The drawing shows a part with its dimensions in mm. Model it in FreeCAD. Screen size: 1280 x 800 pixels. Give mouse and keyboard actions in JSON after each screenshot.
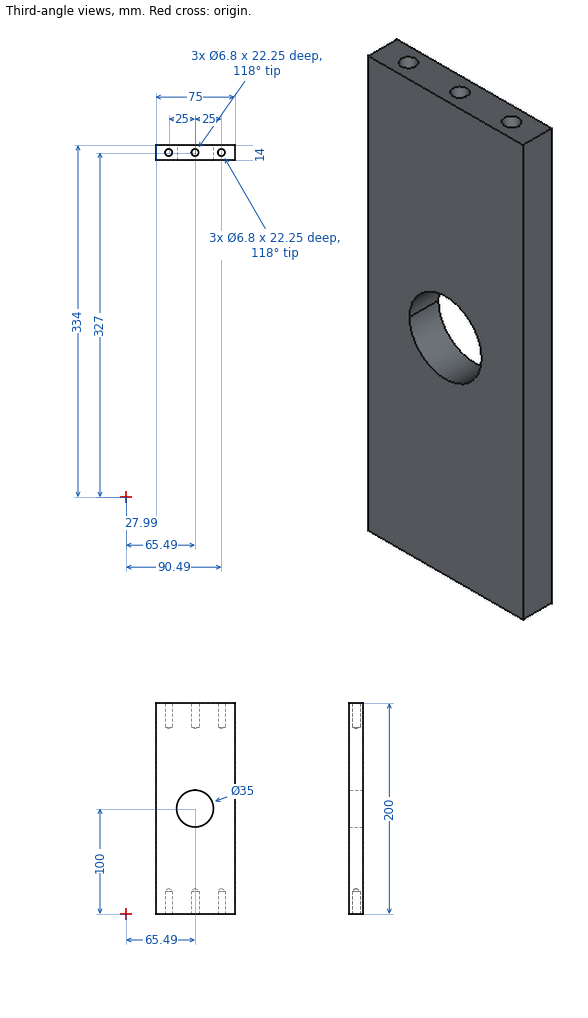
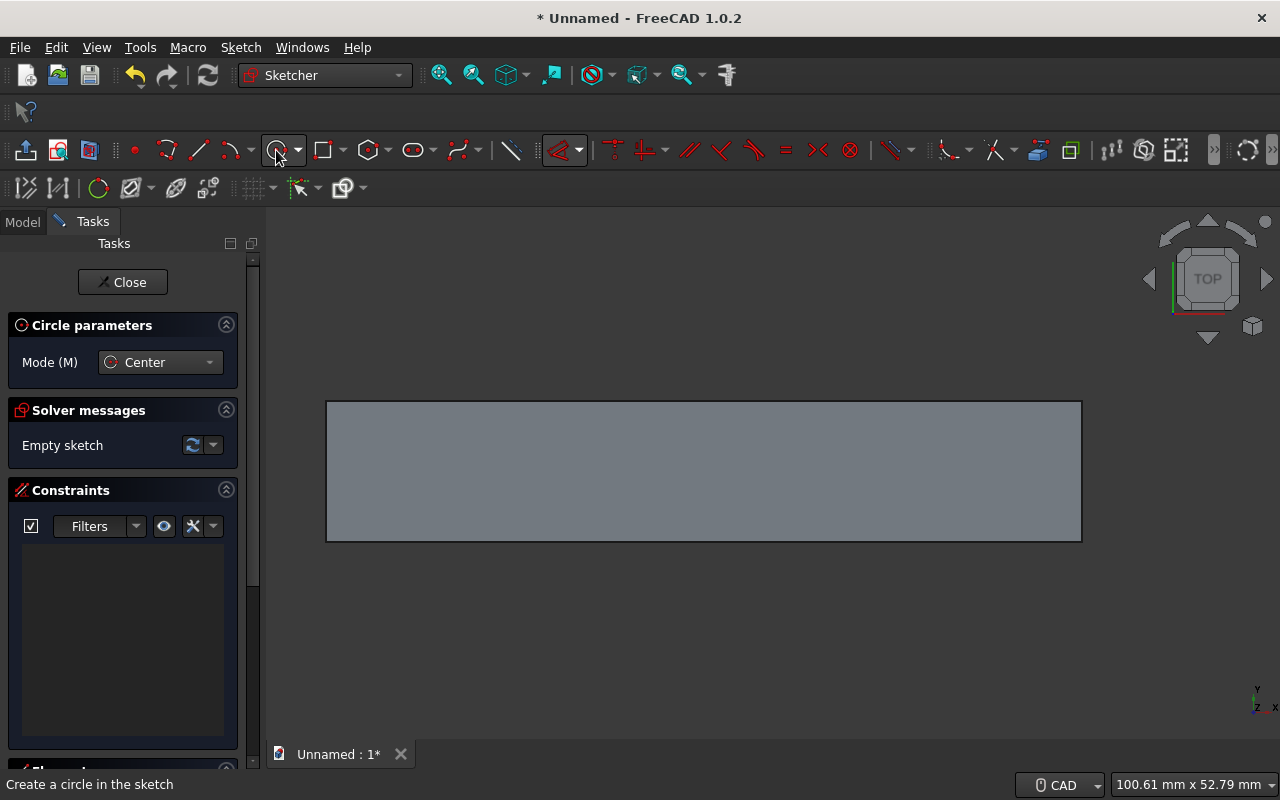
{"action": "left_click", "coordinate": [704, 471]}
{"action": "mouse_move", "coordinate": [728, 447]}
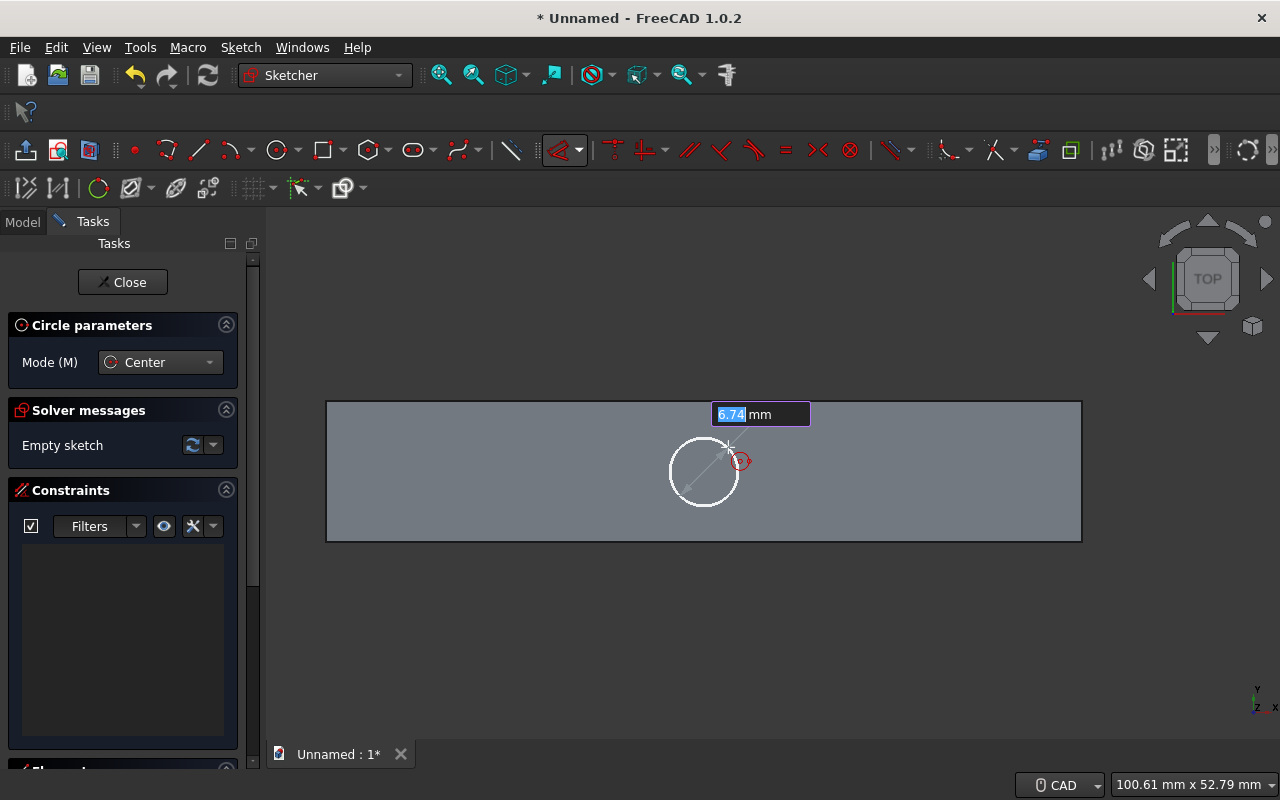
{"action": "type", "text": "6.8"}
{"action": "key", "text": "Return"}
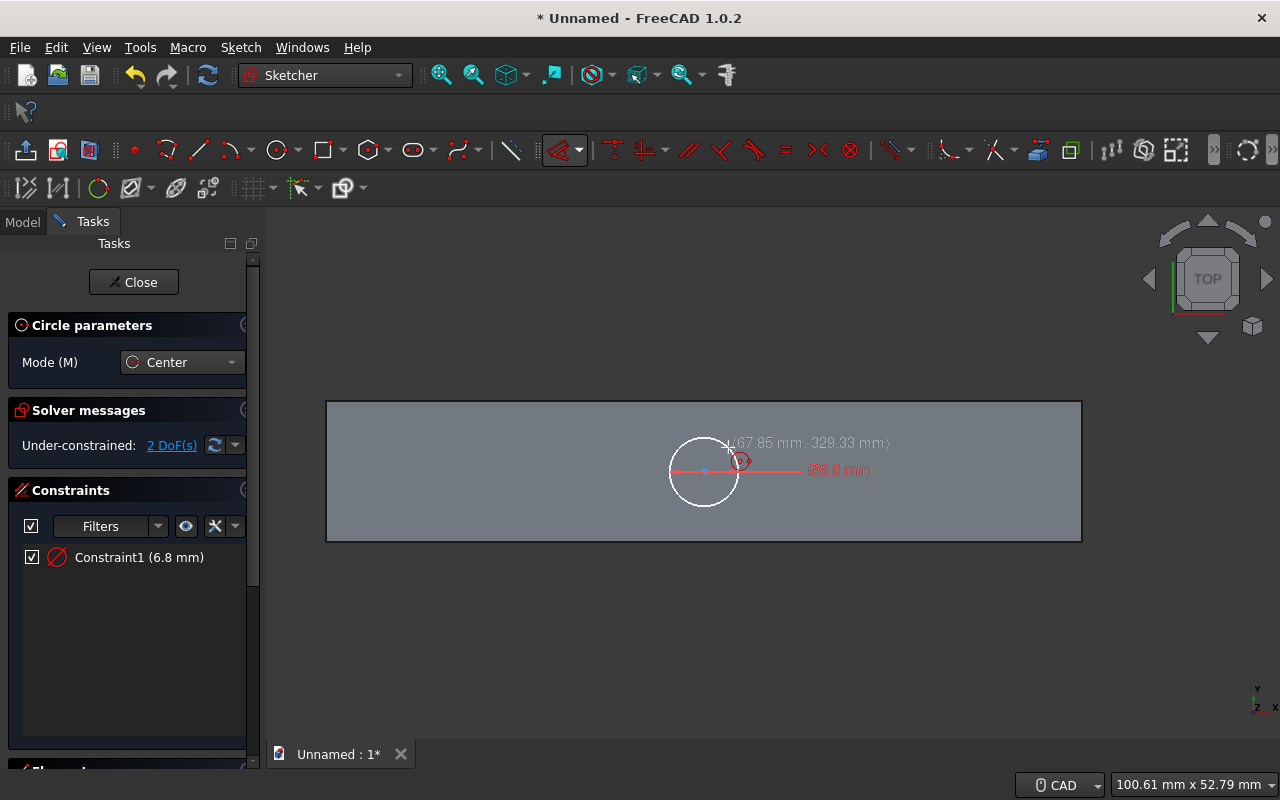
{"action": "left_click", "coordinate": [452, 471]}
{"action": "mouse_move", "coordinate": [476, 447]}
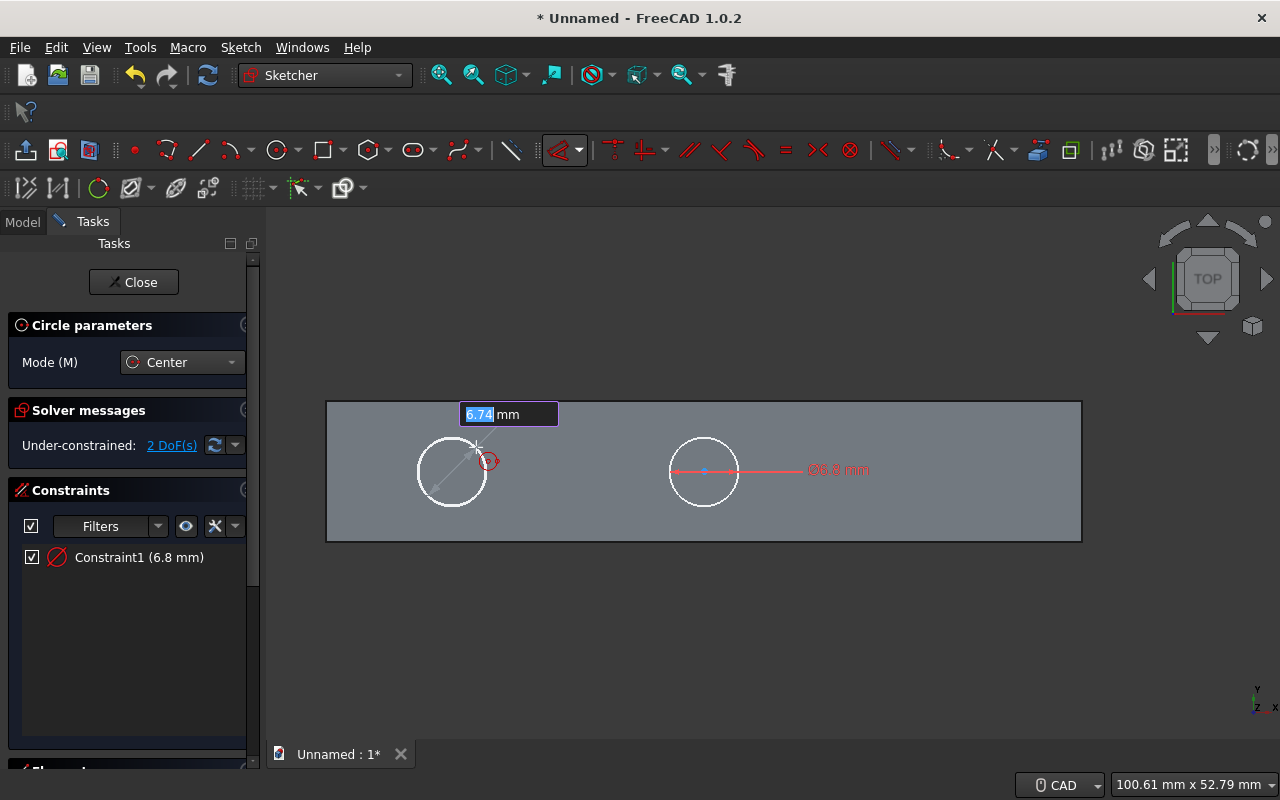
{"action": "type", "text": "6.8"}
{"action": "key", "text": "Return"}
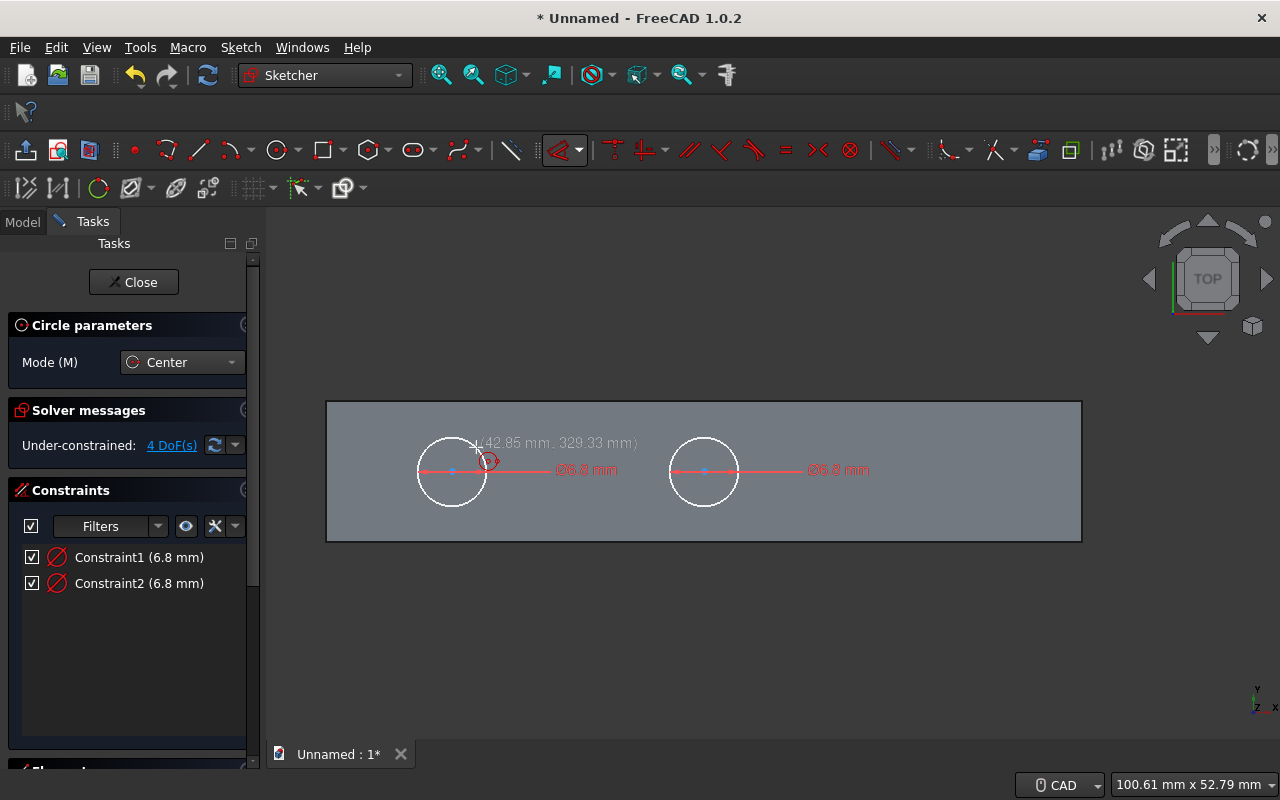
{"action": "left_click", "coordinate": [956, 471]}
{"action": "mouse_move", "coordinate": [980, 447]}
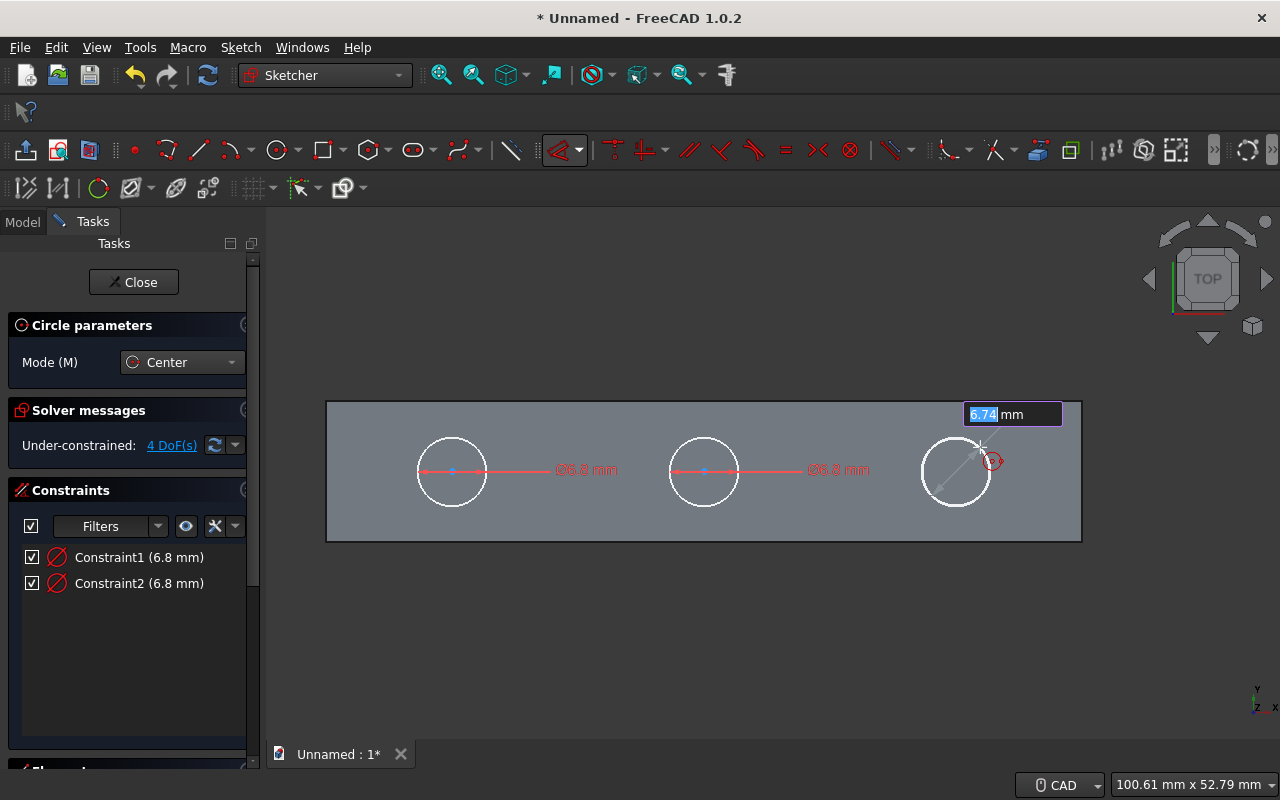
{"action": "type", "text": "6.8"}
{"action": "key", "text": "Return"}
{"action": "key", "text": "Escape"}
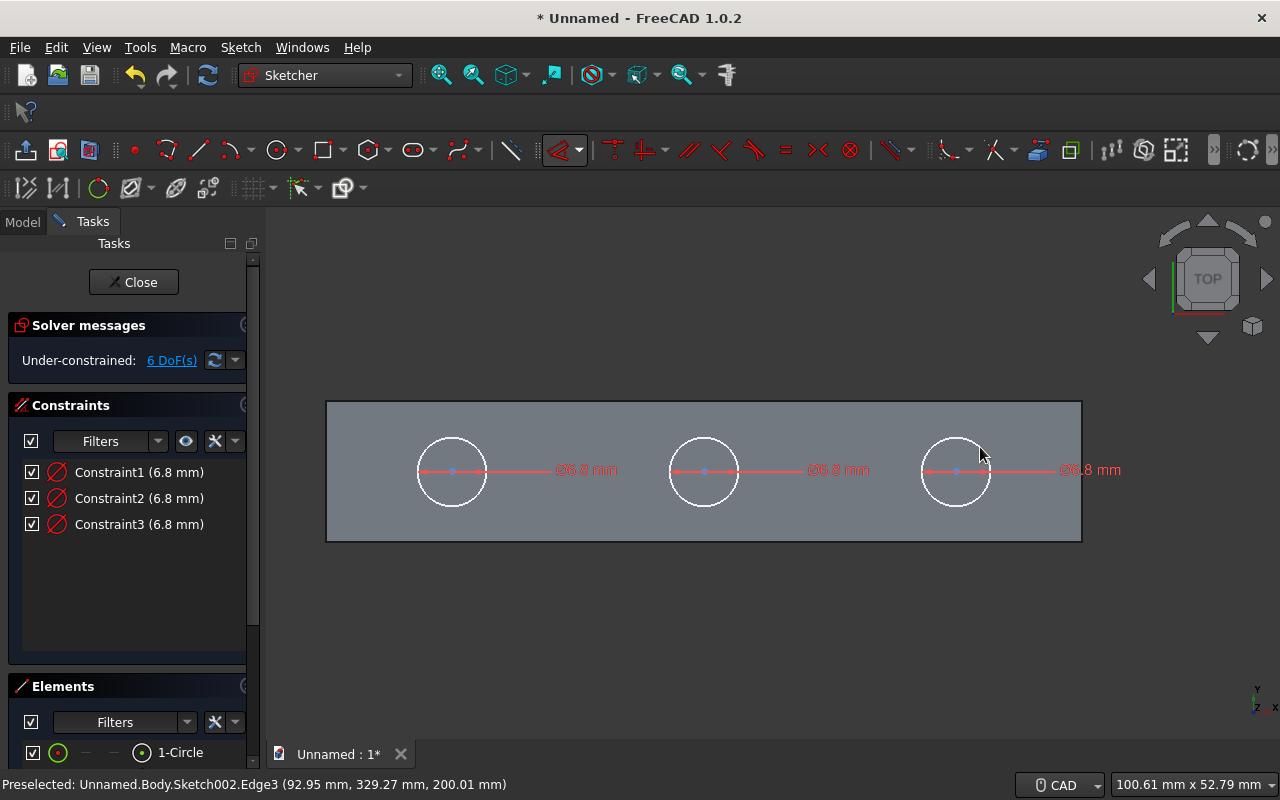
{"action": "left_click", "coordinate": [704, 472]}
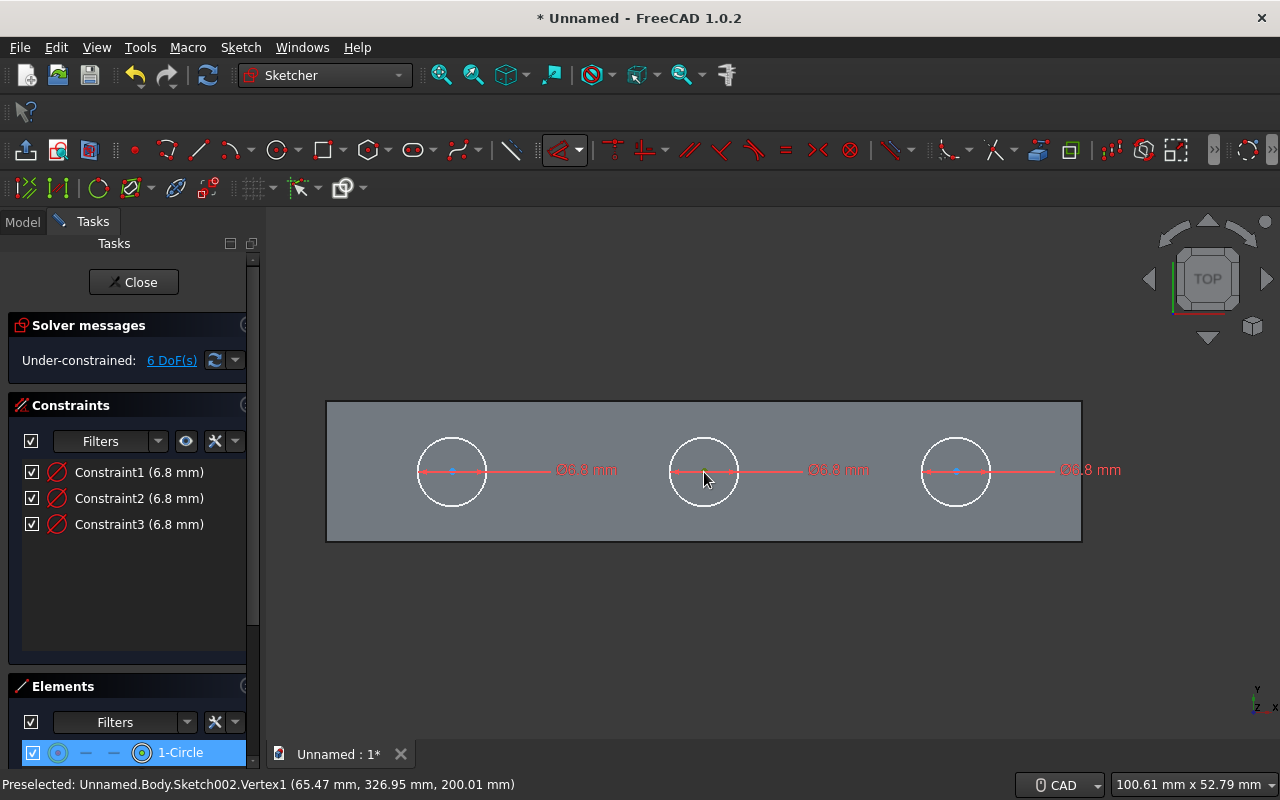
{"action": "left_click", "coordinate": [452, 472]}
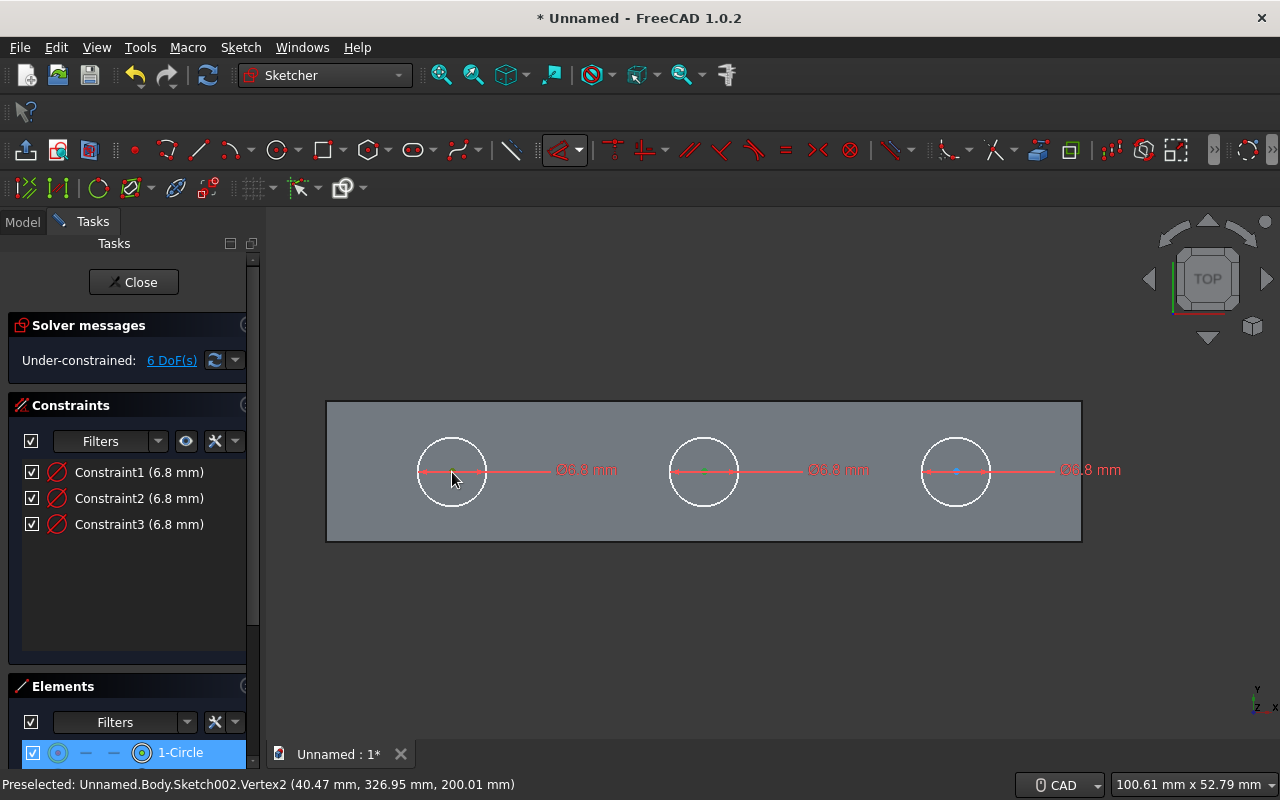
{"action": "key", "text": "h"}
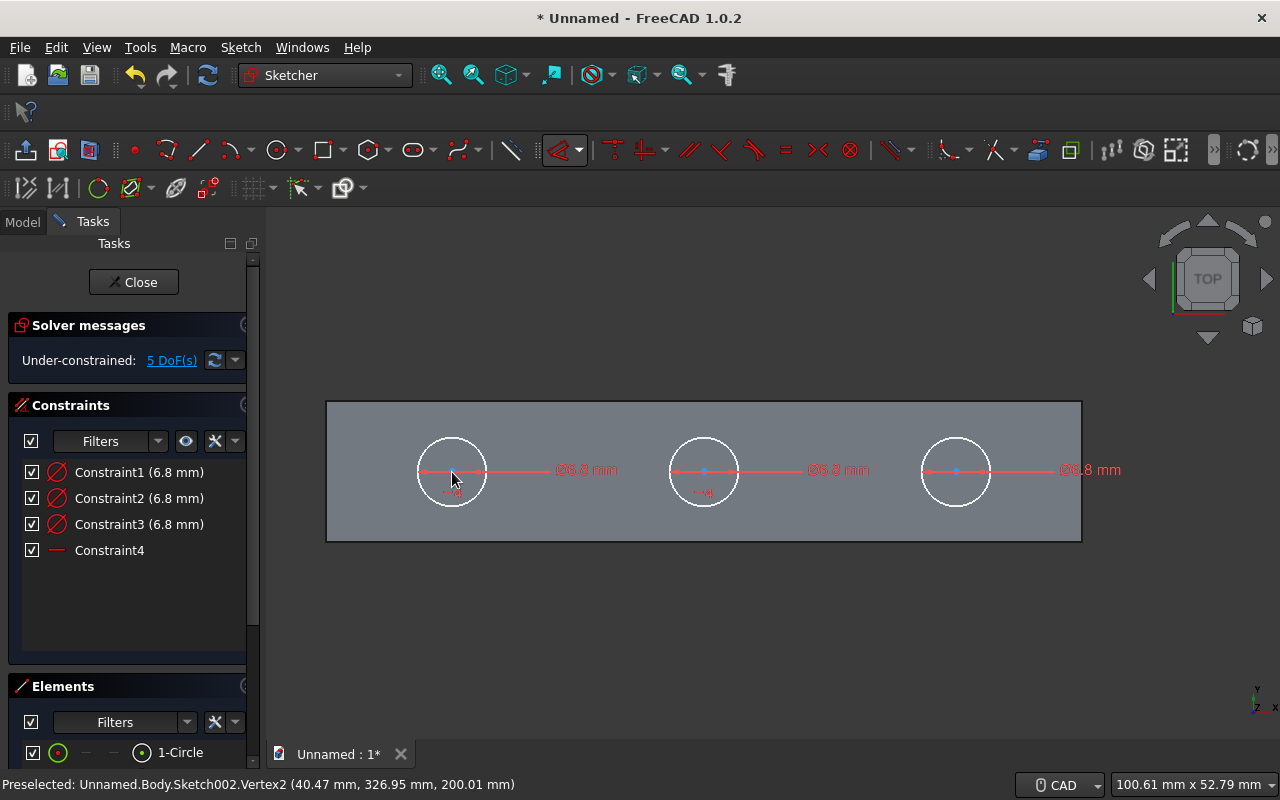
{"action": "left_click", "coordinate": [704, 472]}